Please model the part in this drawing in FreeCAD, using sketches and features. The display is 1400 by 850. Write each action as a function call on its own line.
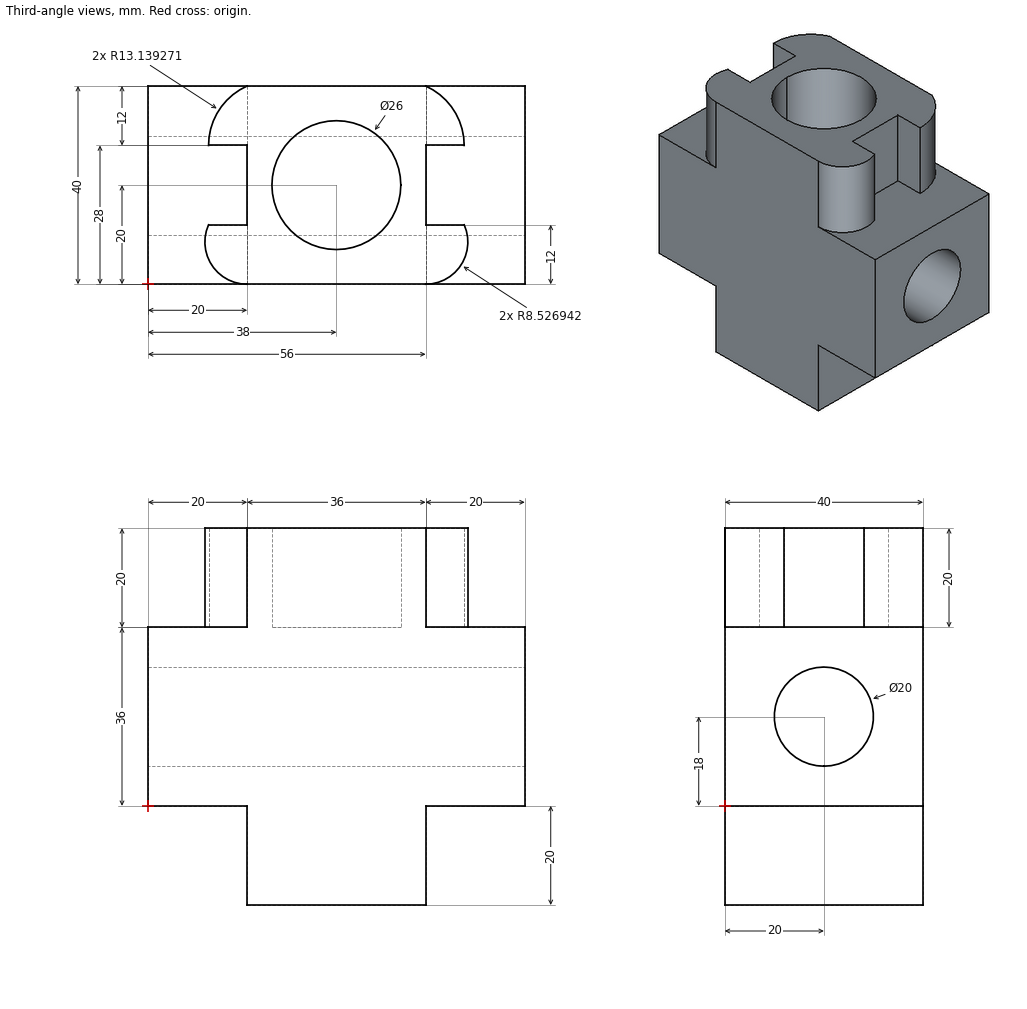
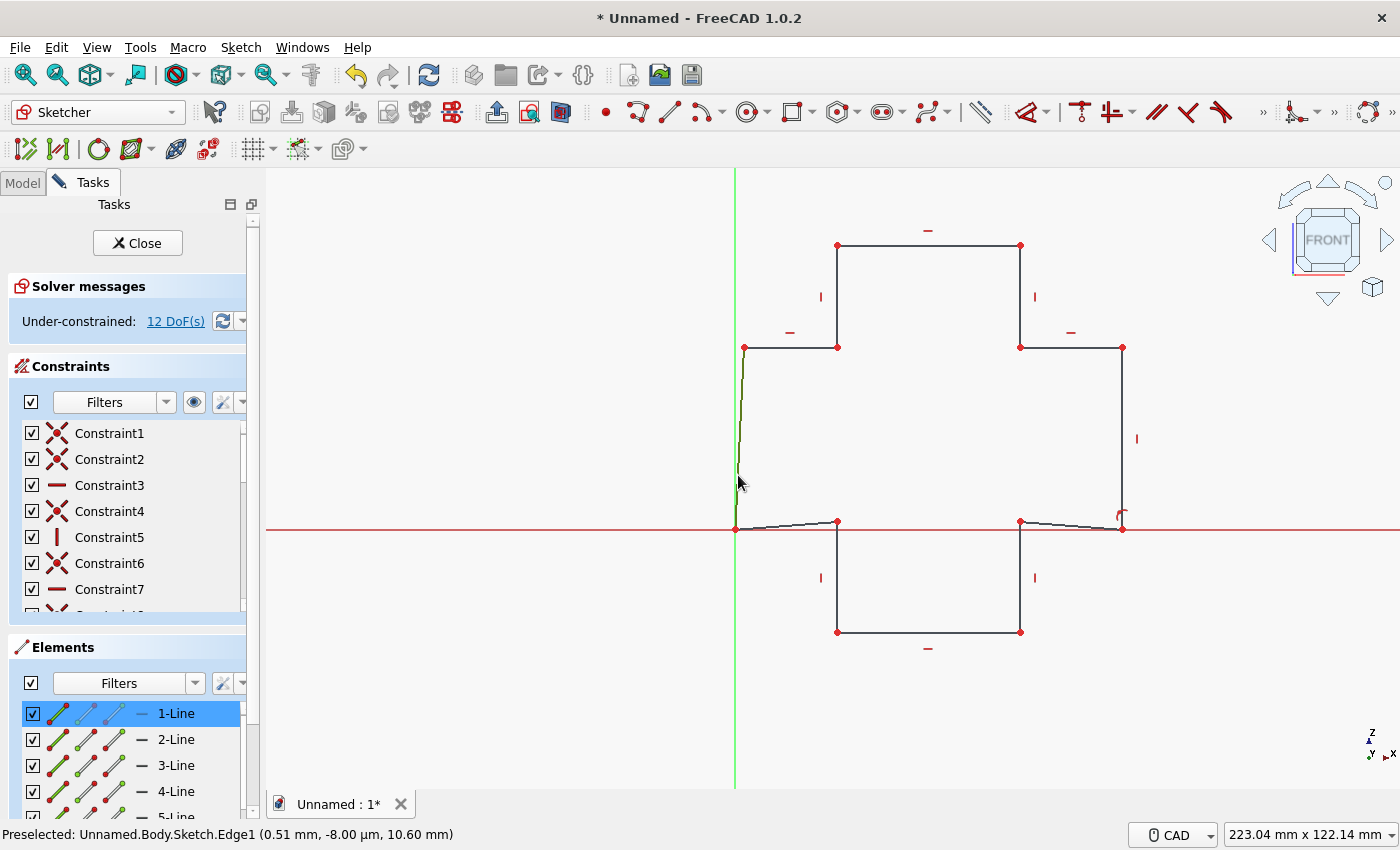
click(1134, 112)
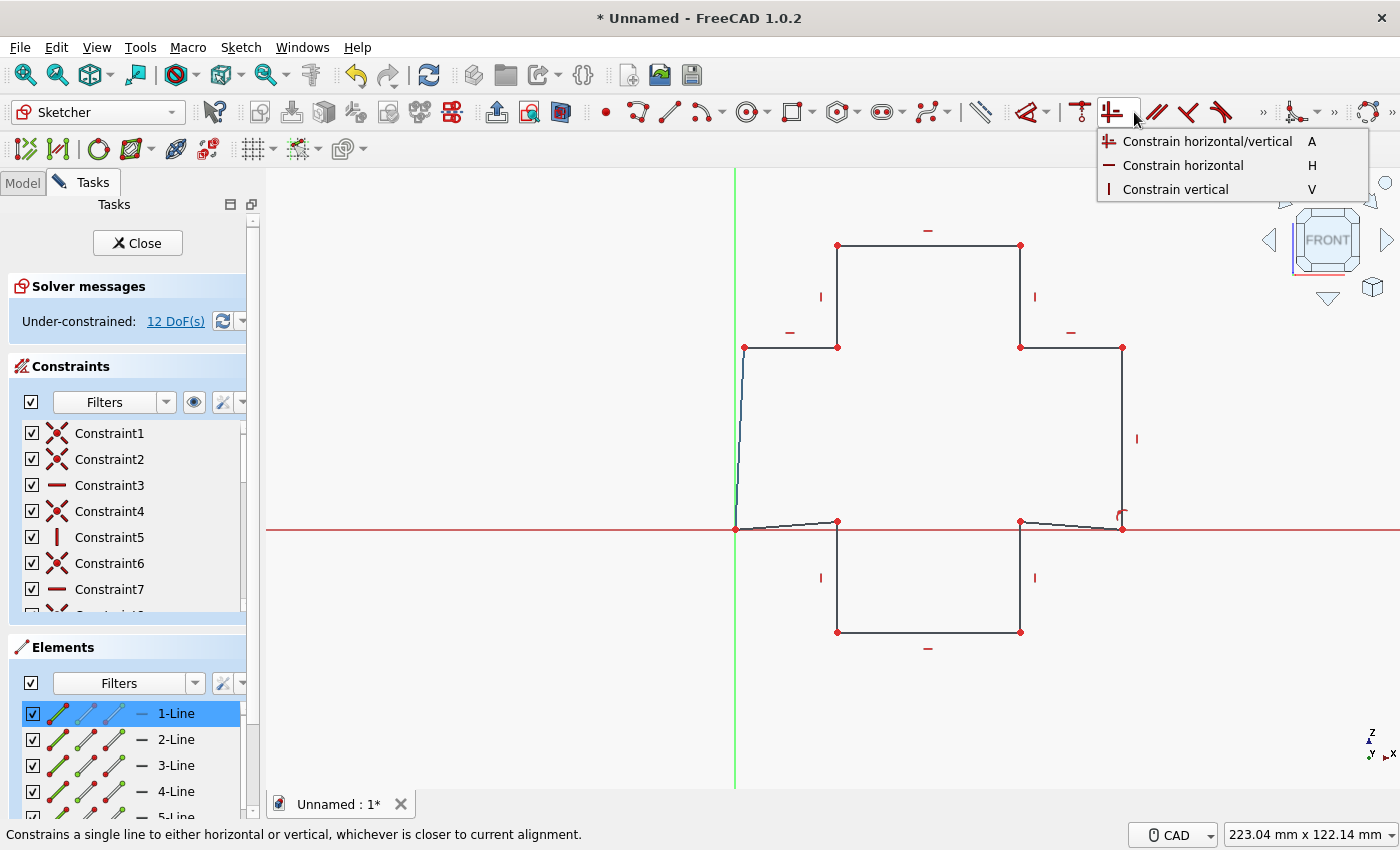
click(1233, 189)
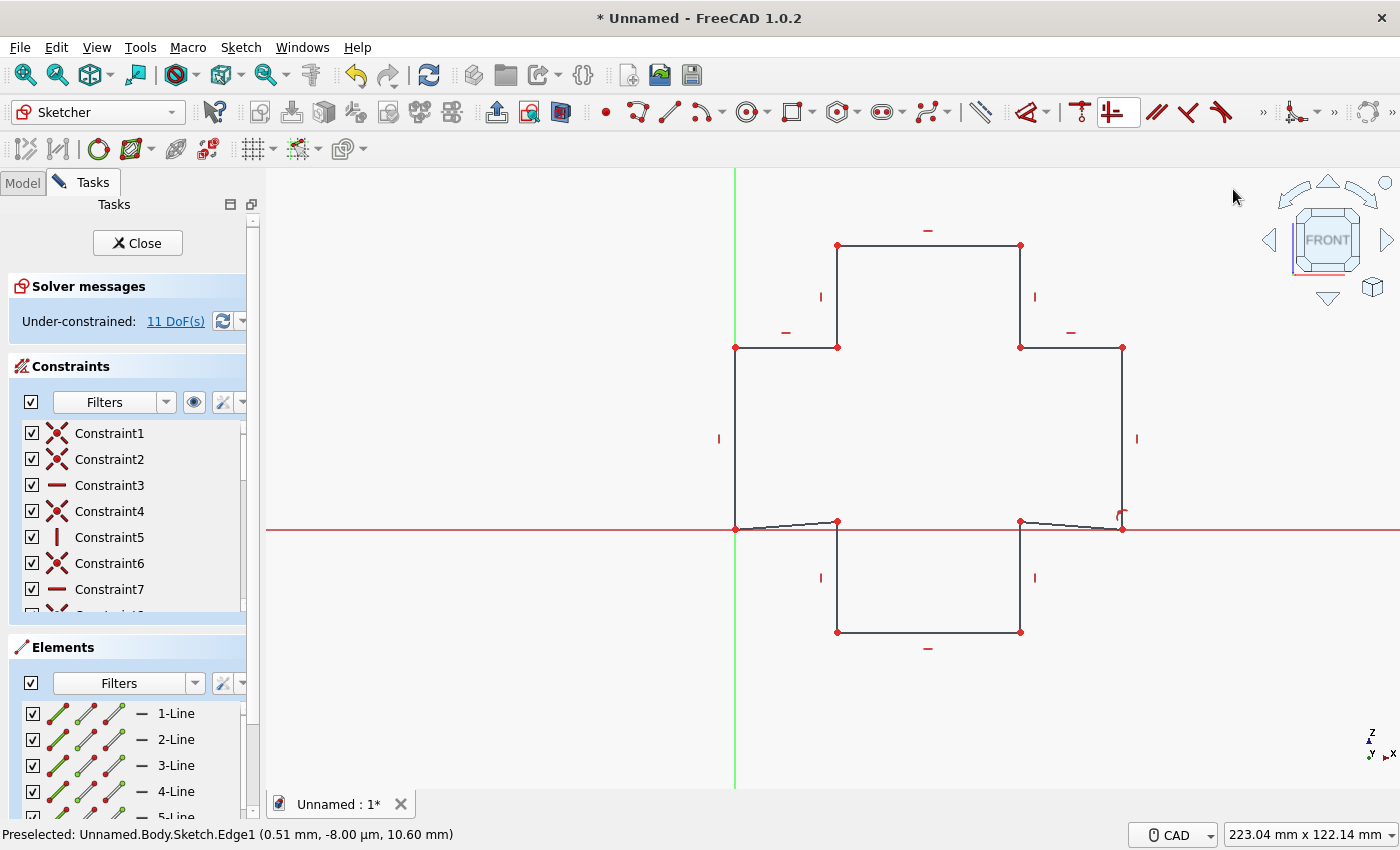
click(1091, 528)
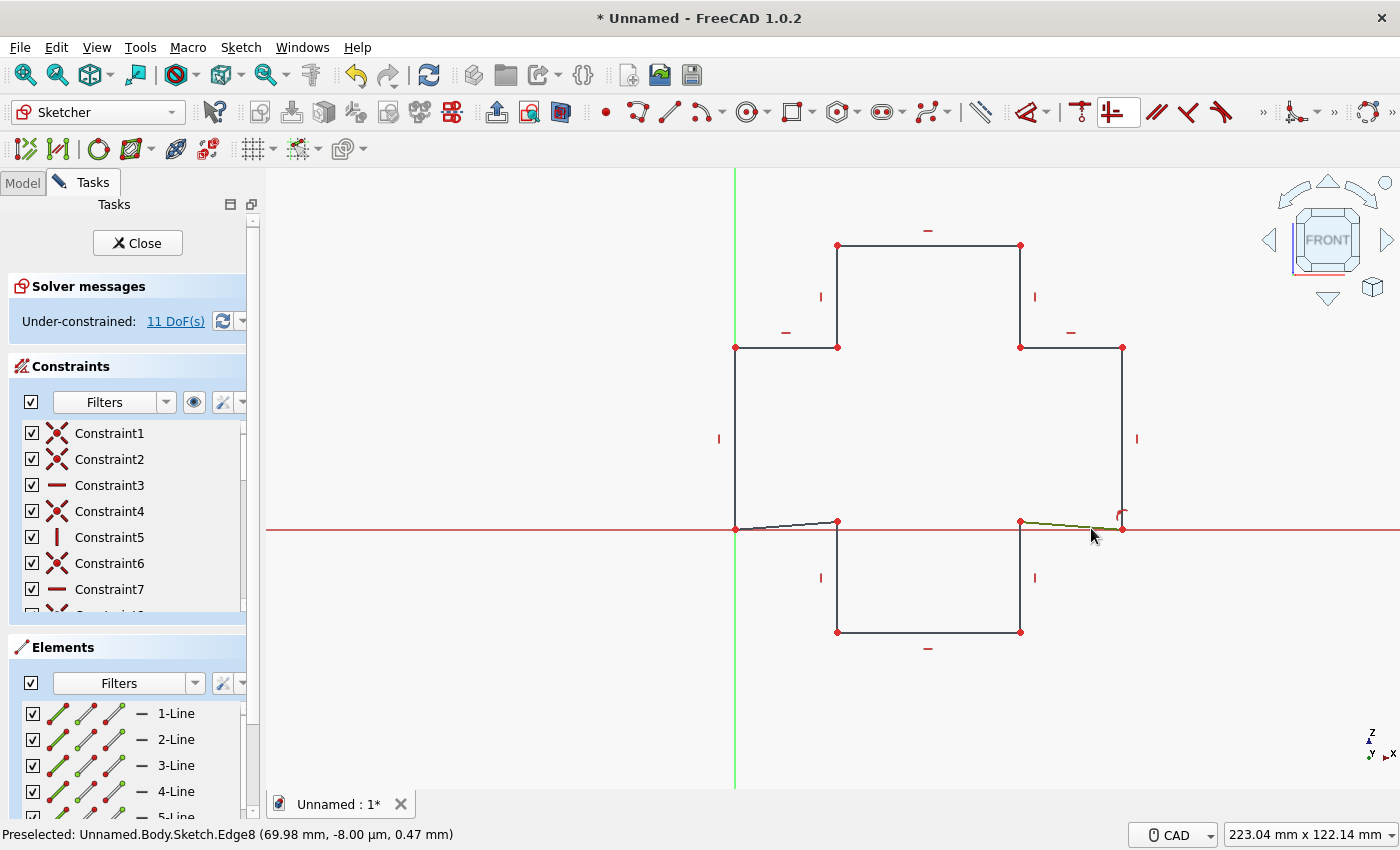
click(1134, 112)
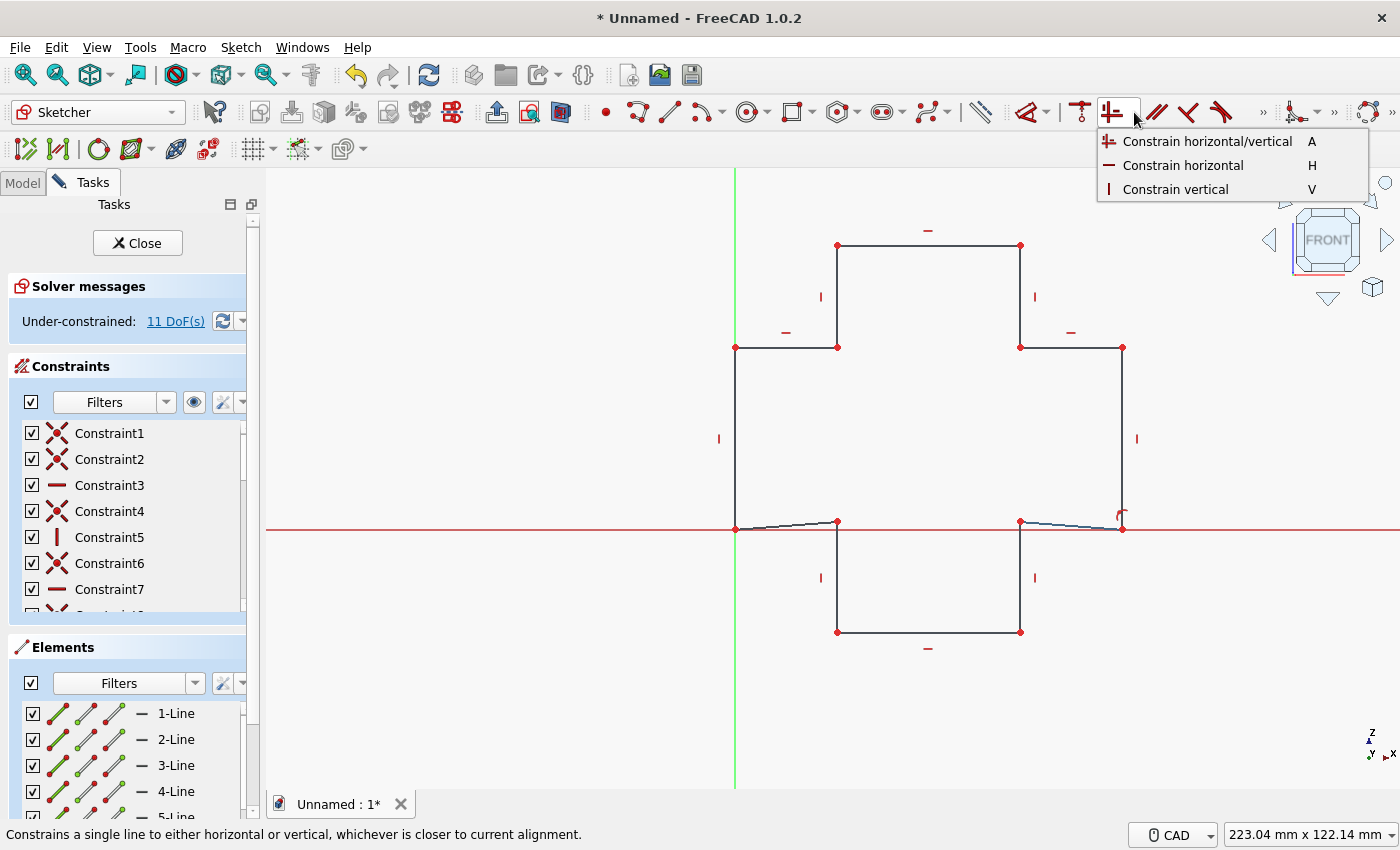
click(1233, 165)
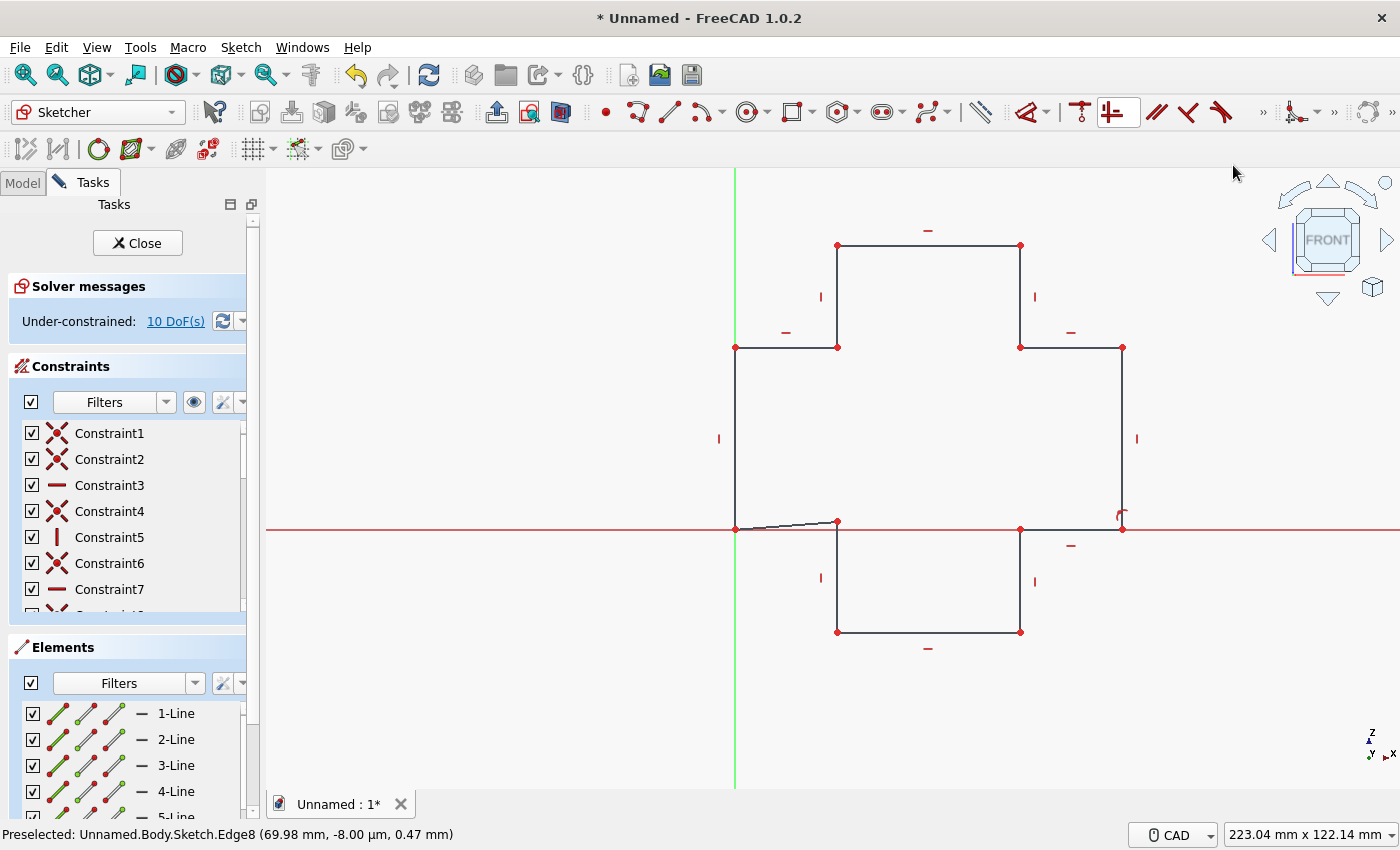
click(766, 528)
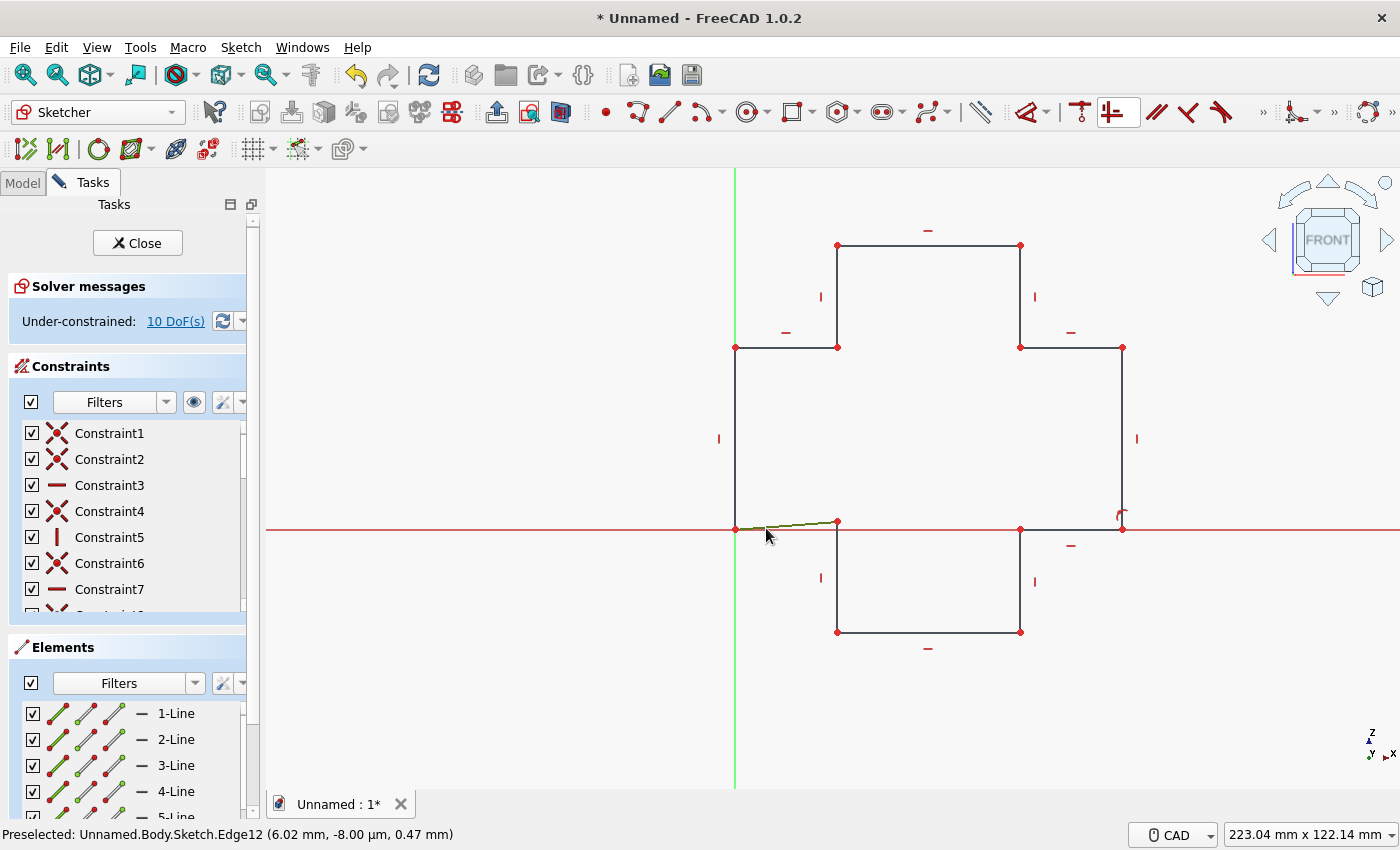
key(h)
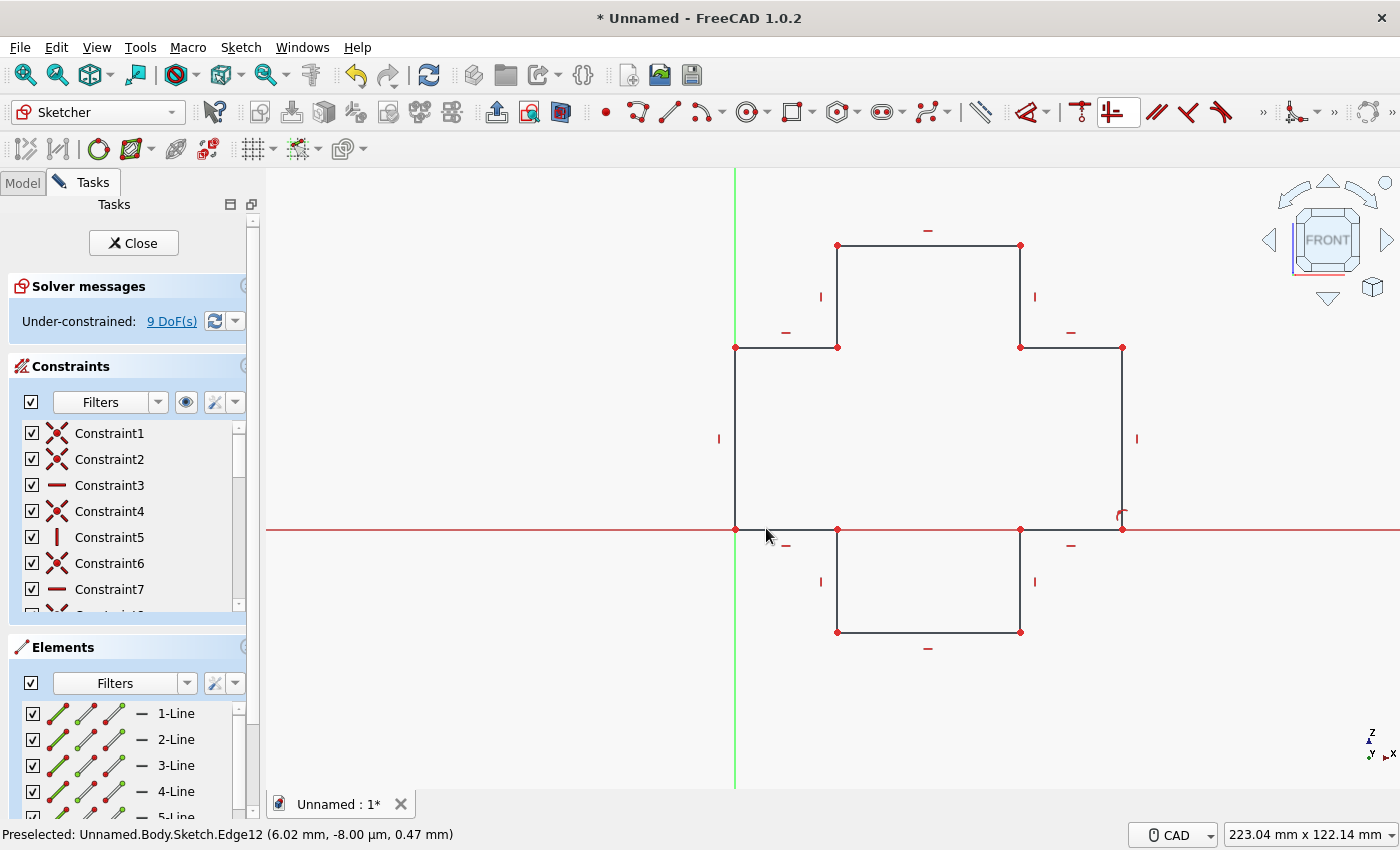
click(1026, 112)